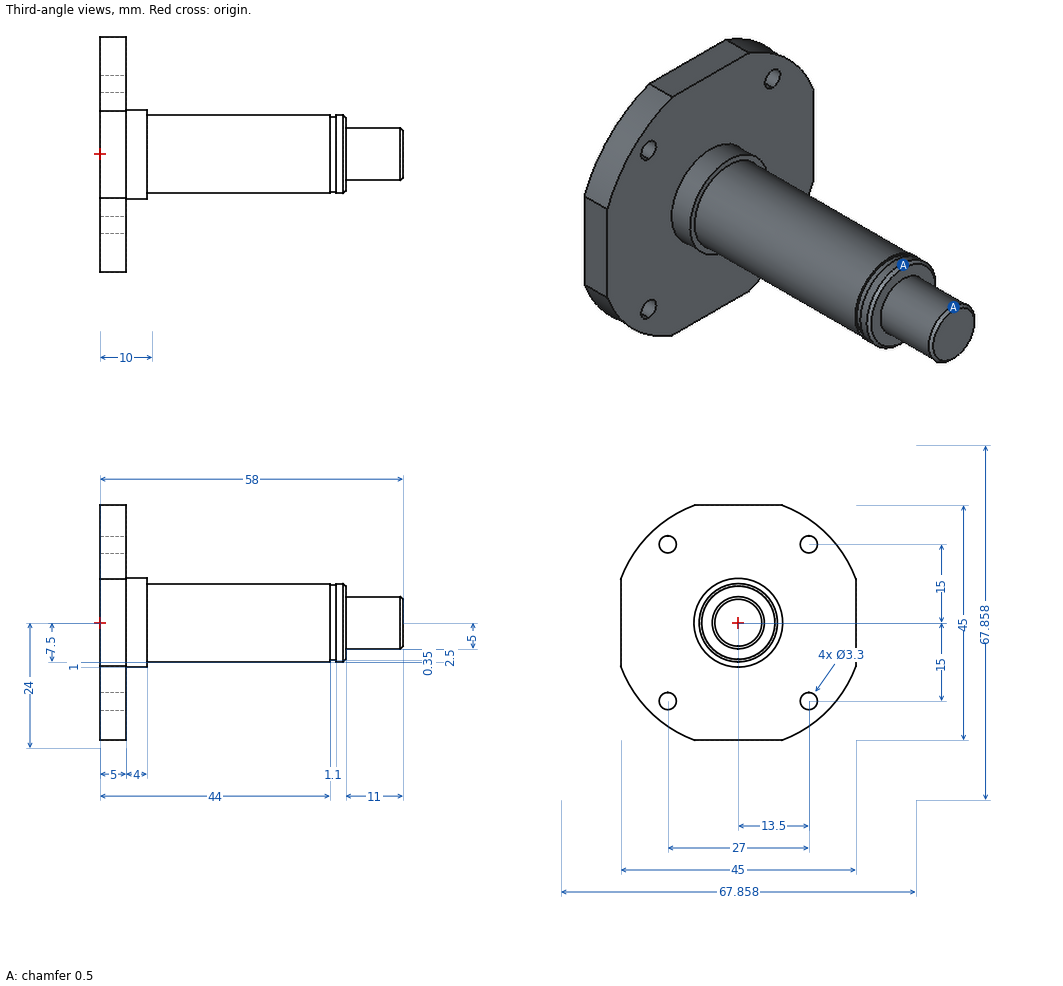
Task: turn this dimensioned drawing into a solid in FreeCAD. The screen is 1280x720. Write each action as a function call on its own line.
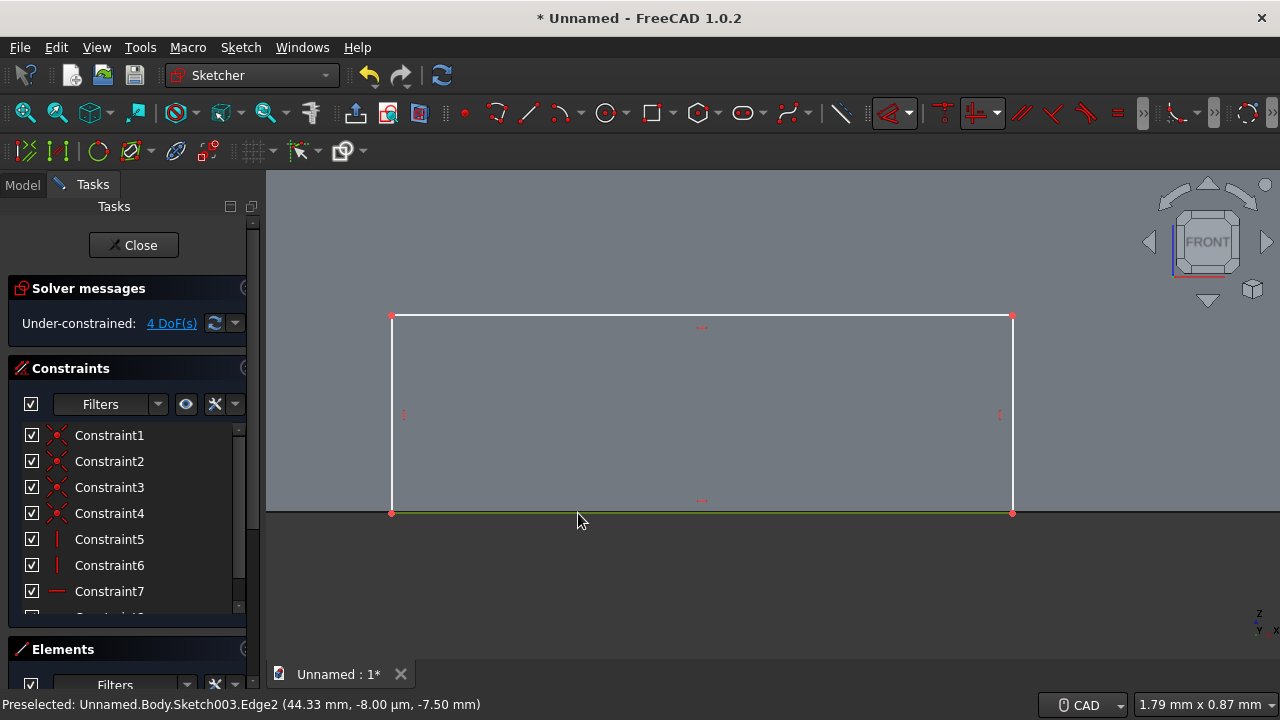
click(912, 114)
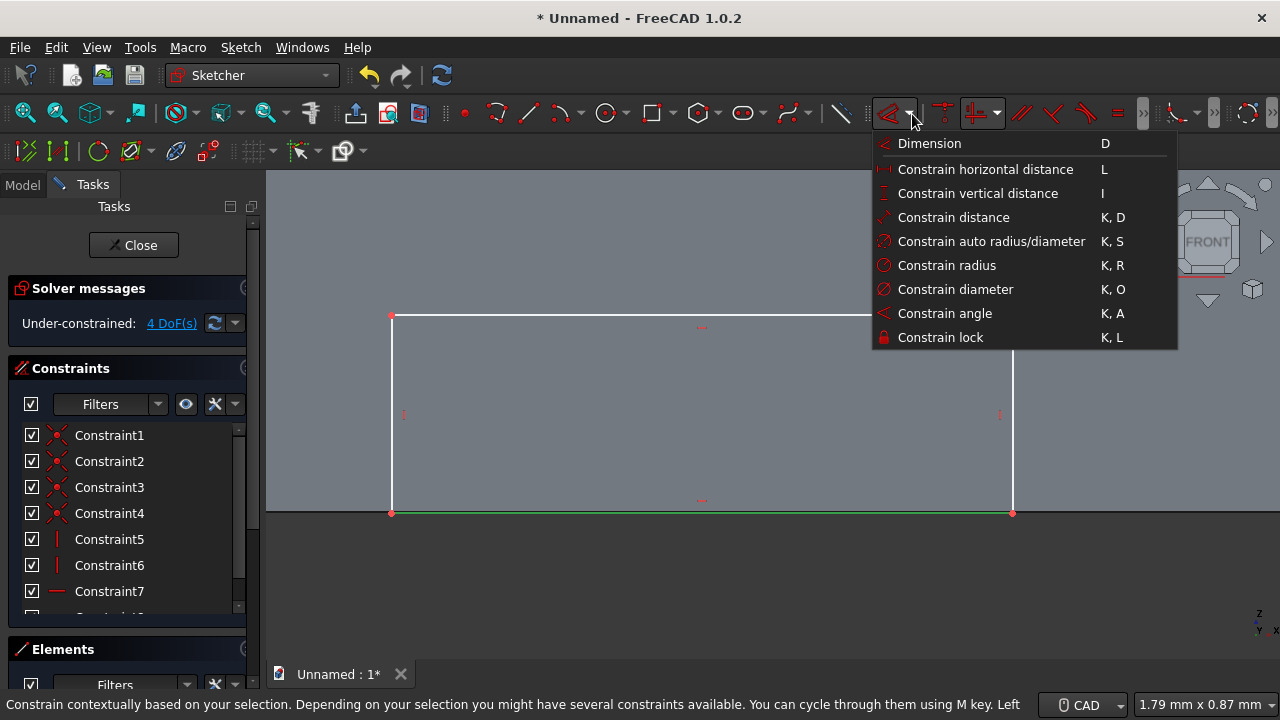
click(1025, 169)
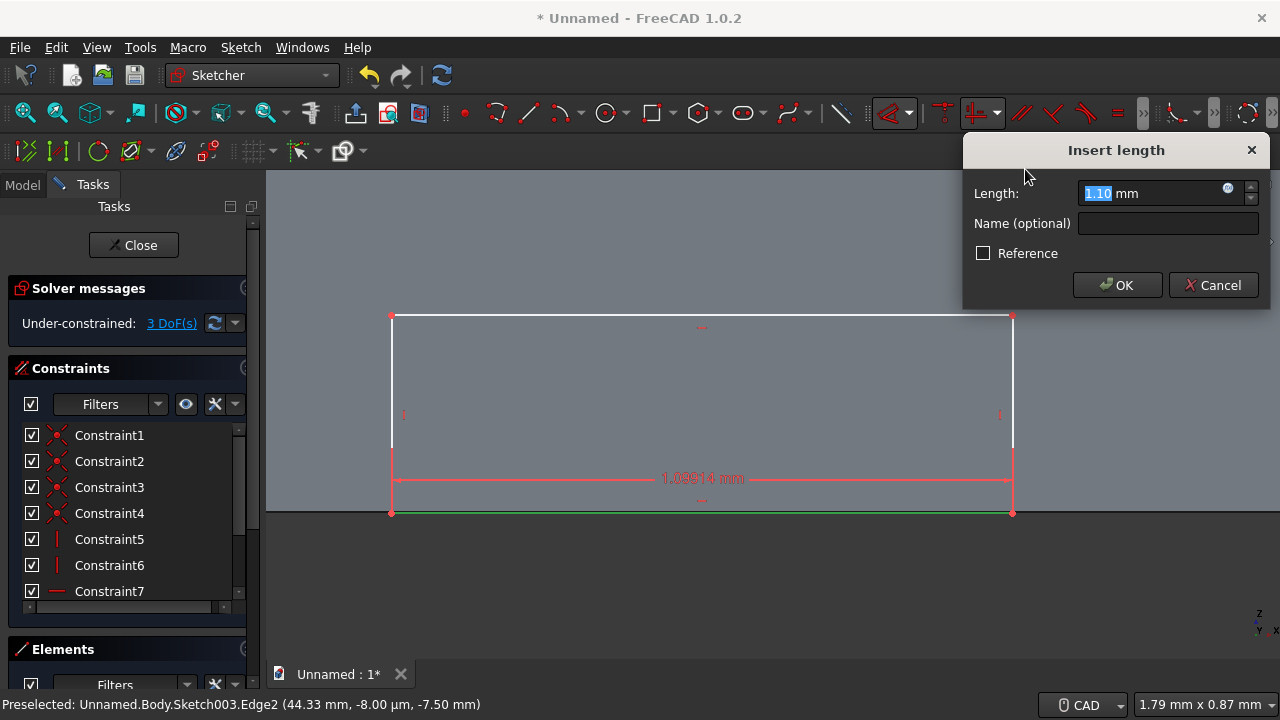
text(1.1)
key(Return)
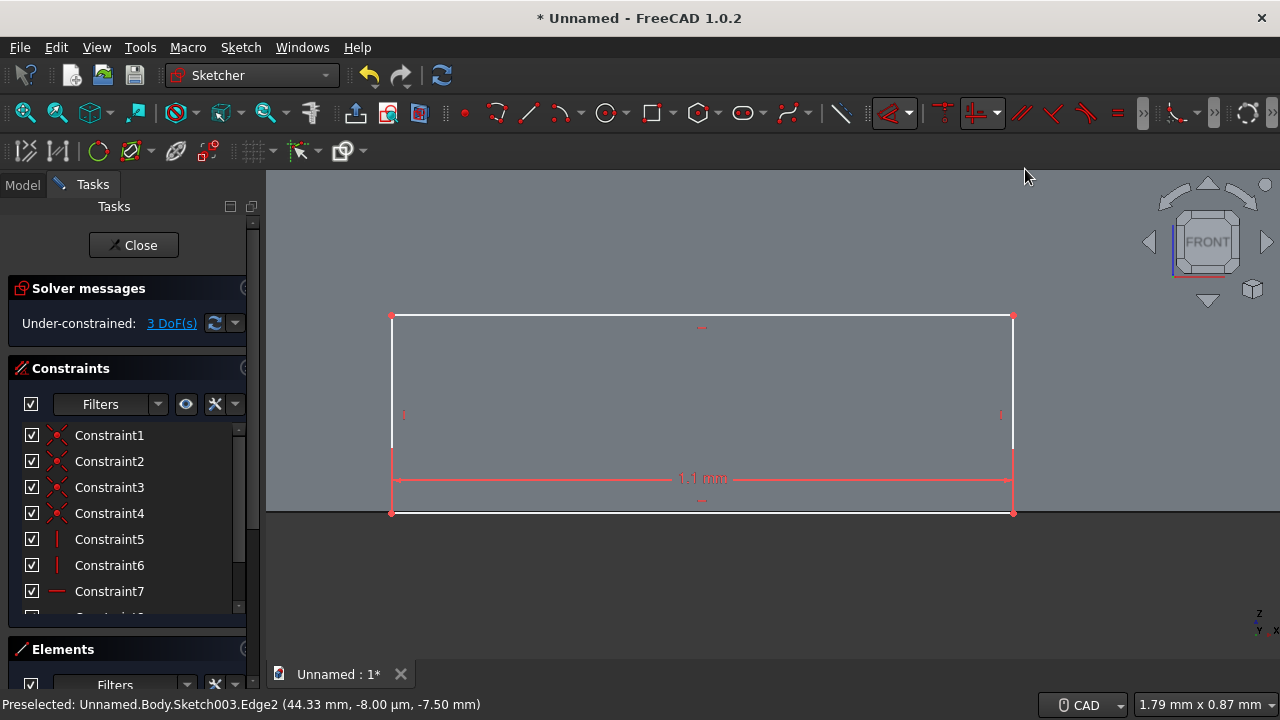
click(392, 315)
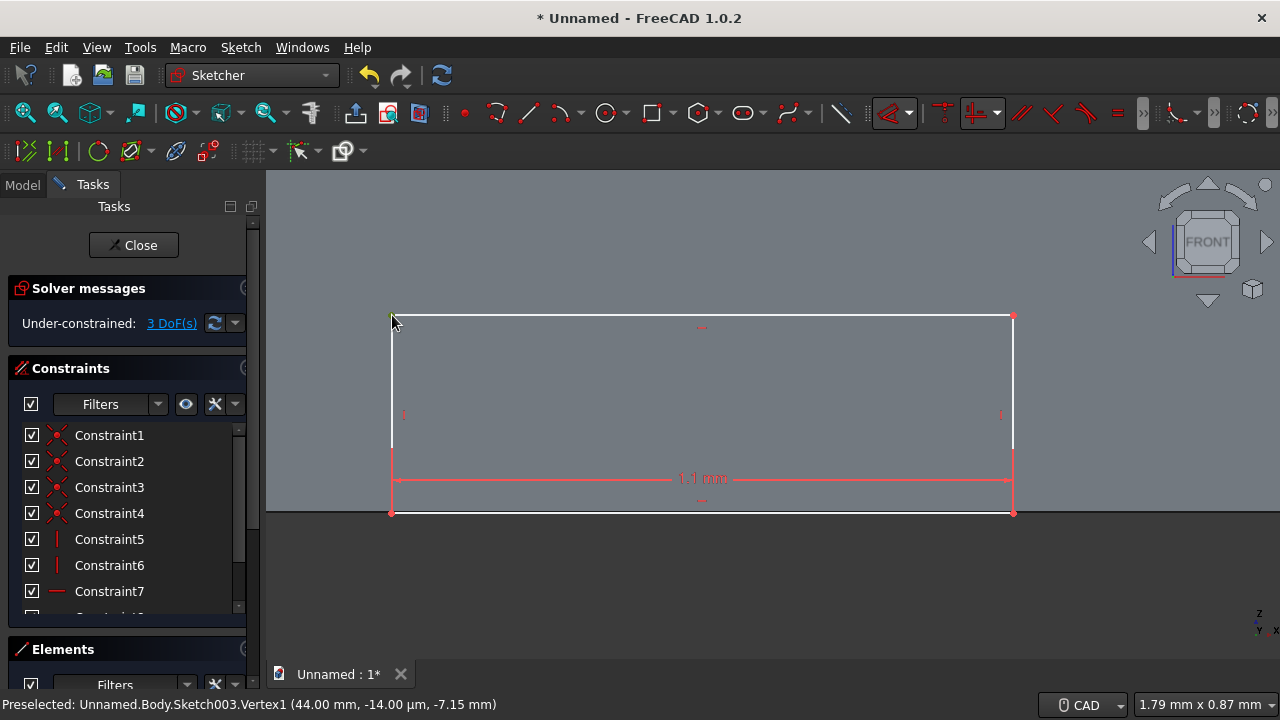
key(l)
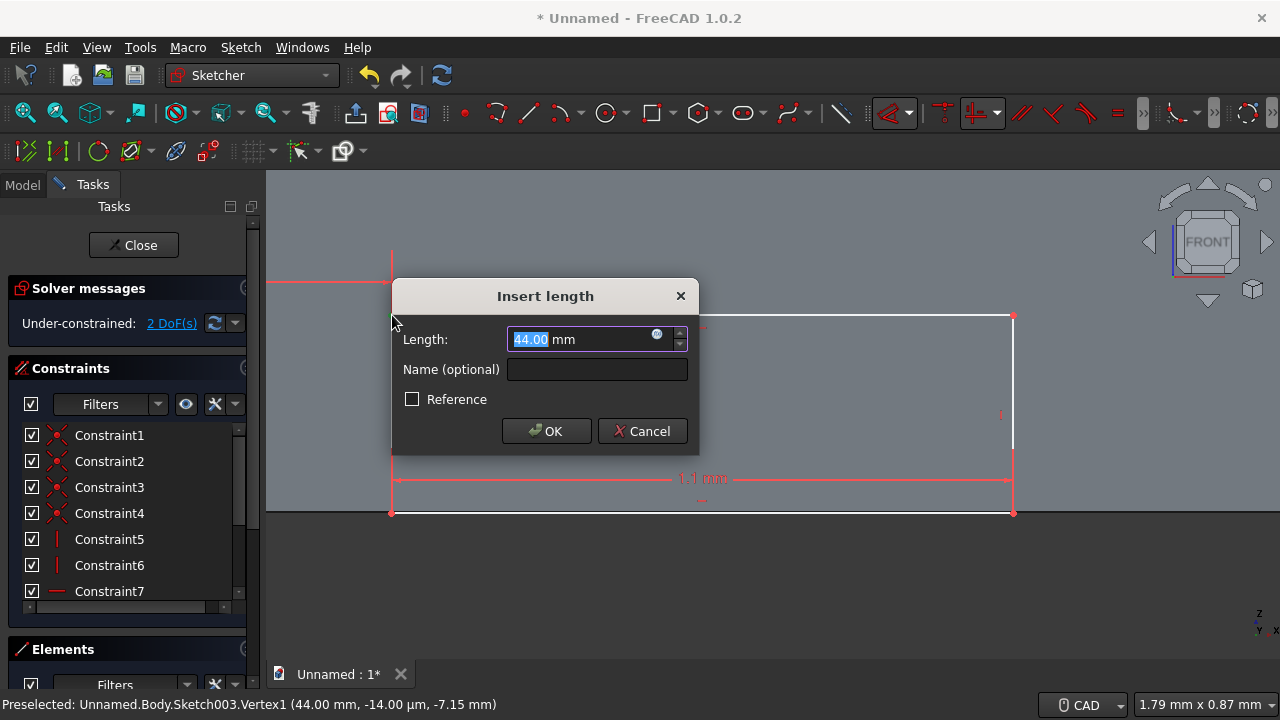
text(44)
key(Return)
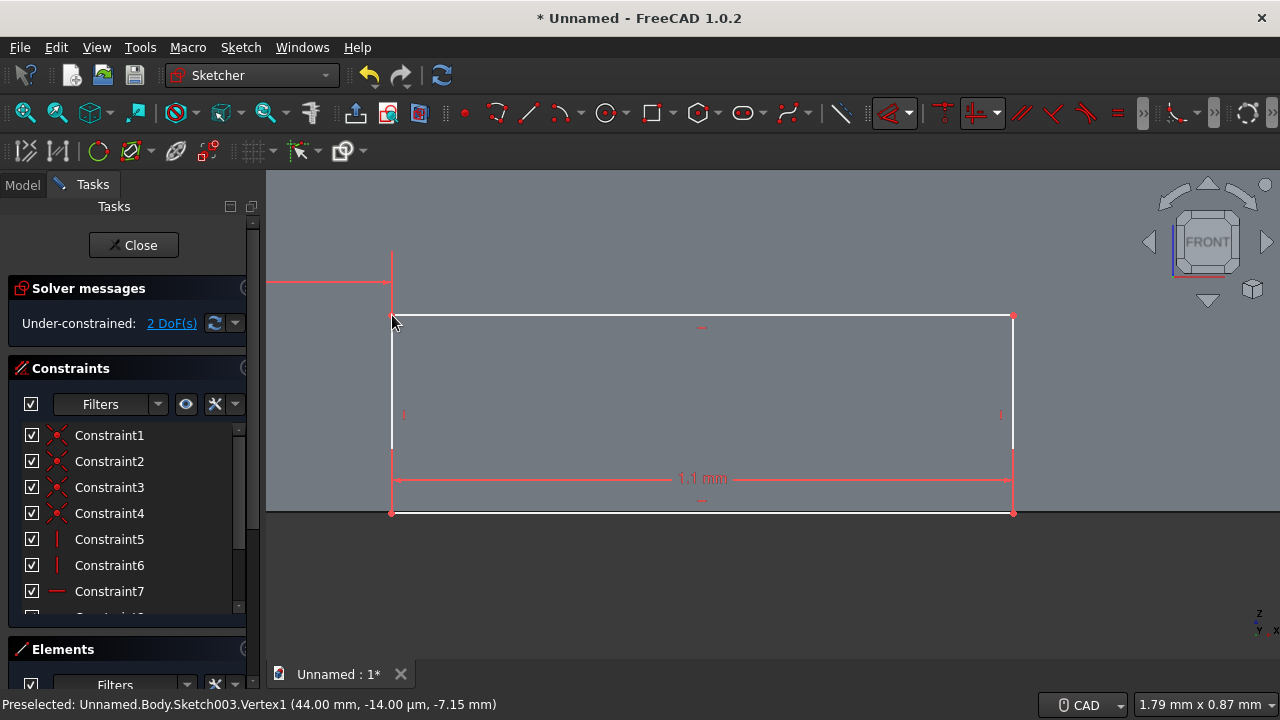
click(392, 374)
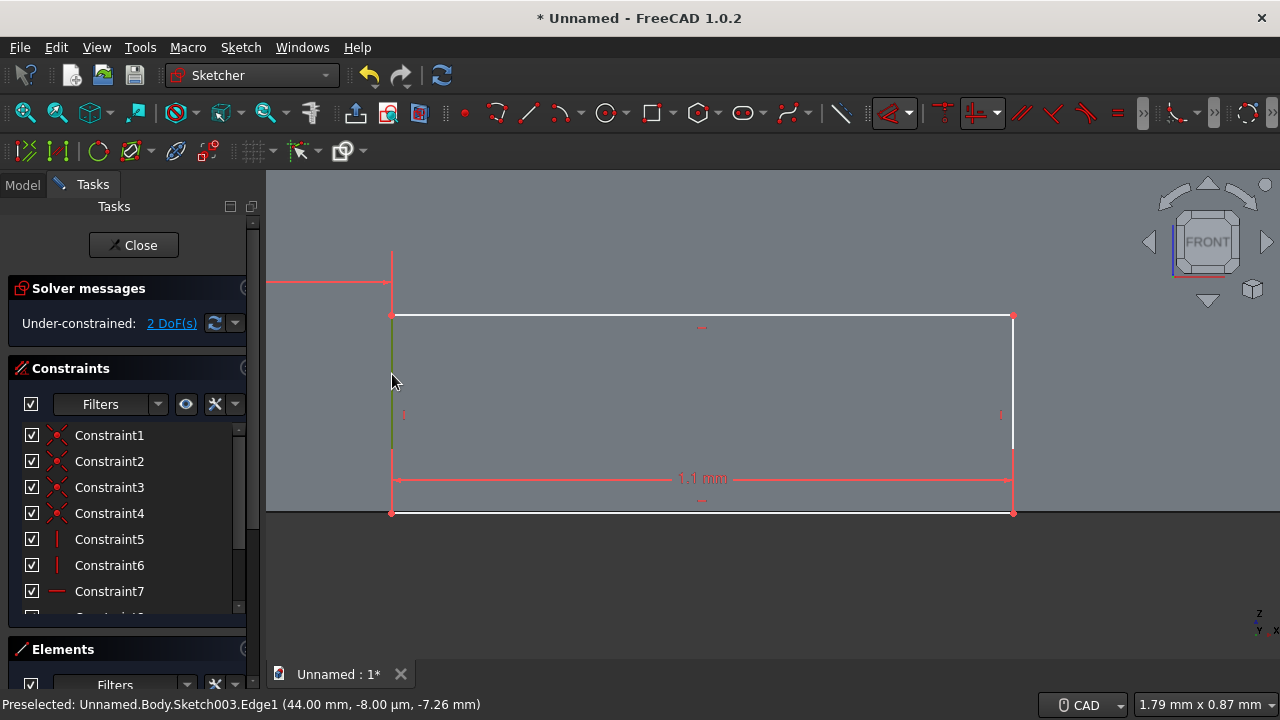
click(912, 114)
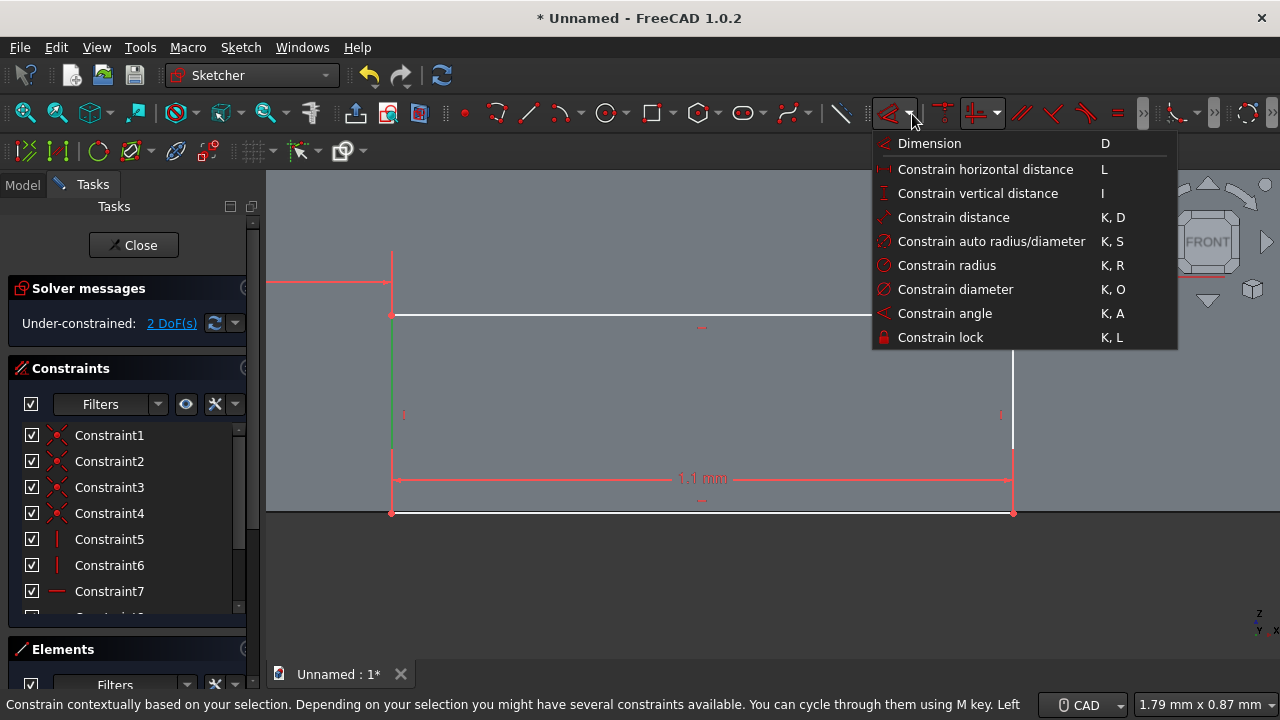
click(1025, 193)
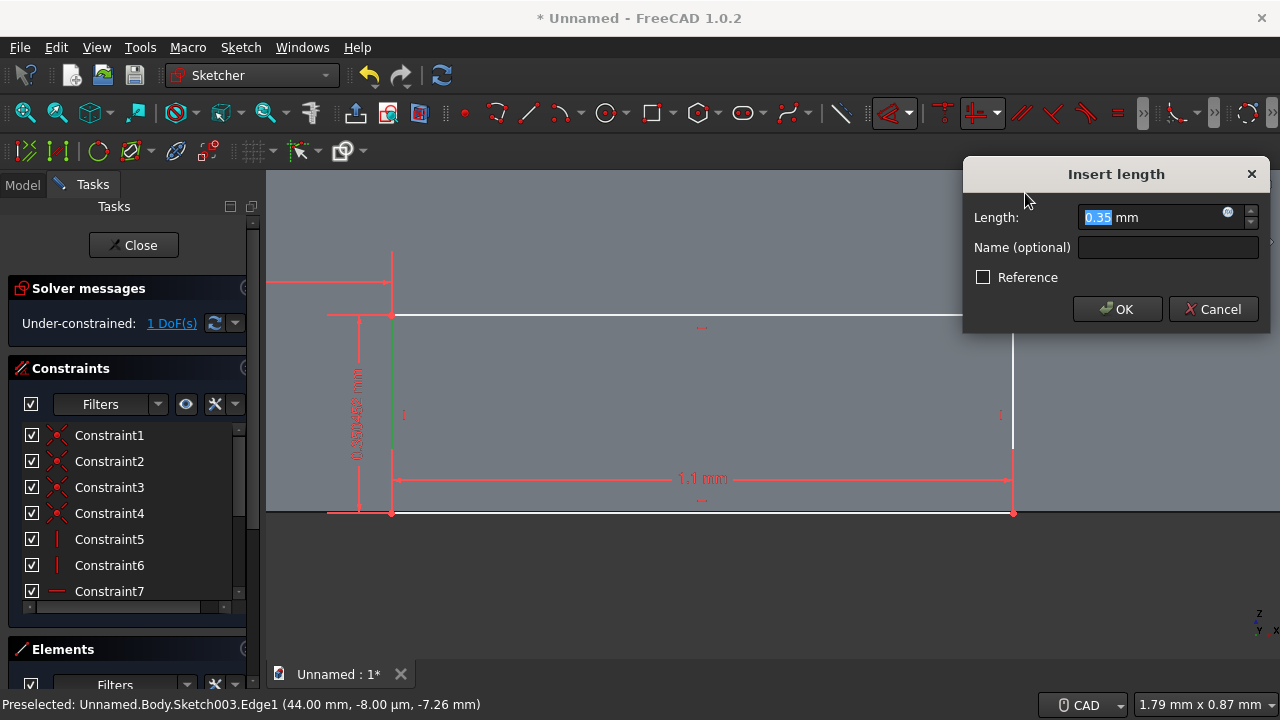
text(0.35)
key(Return)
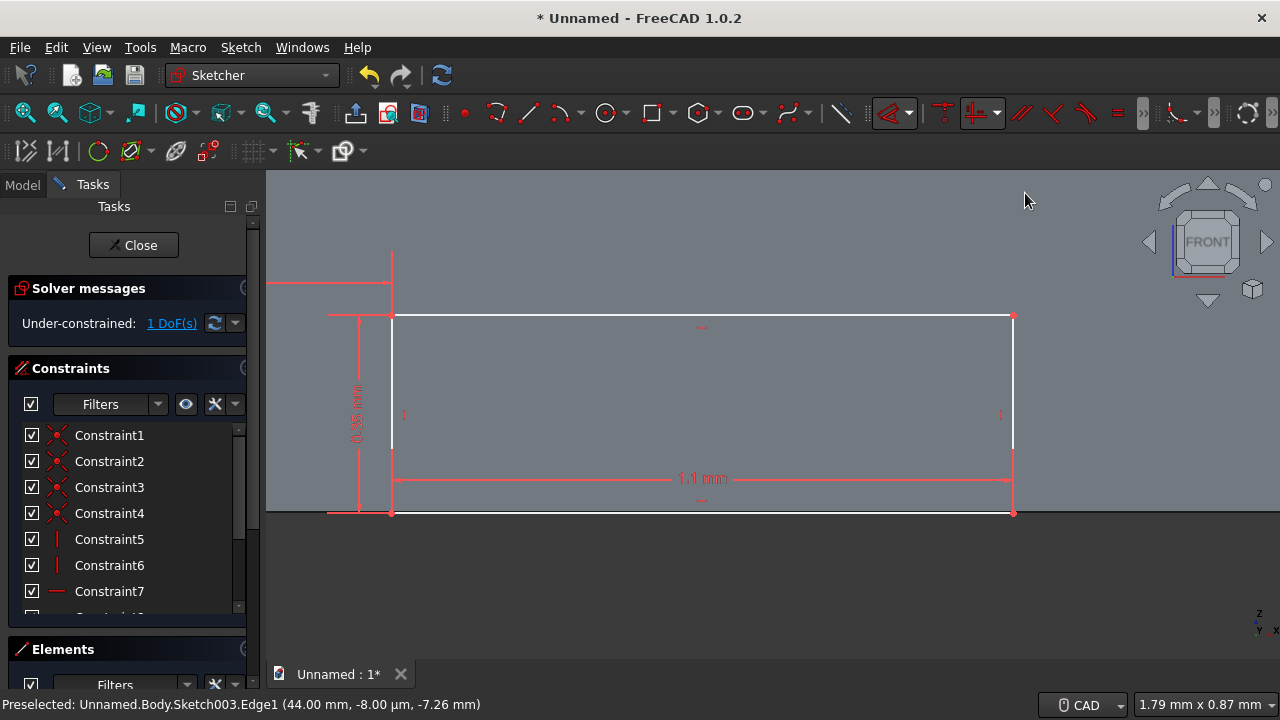
click(392, 513)